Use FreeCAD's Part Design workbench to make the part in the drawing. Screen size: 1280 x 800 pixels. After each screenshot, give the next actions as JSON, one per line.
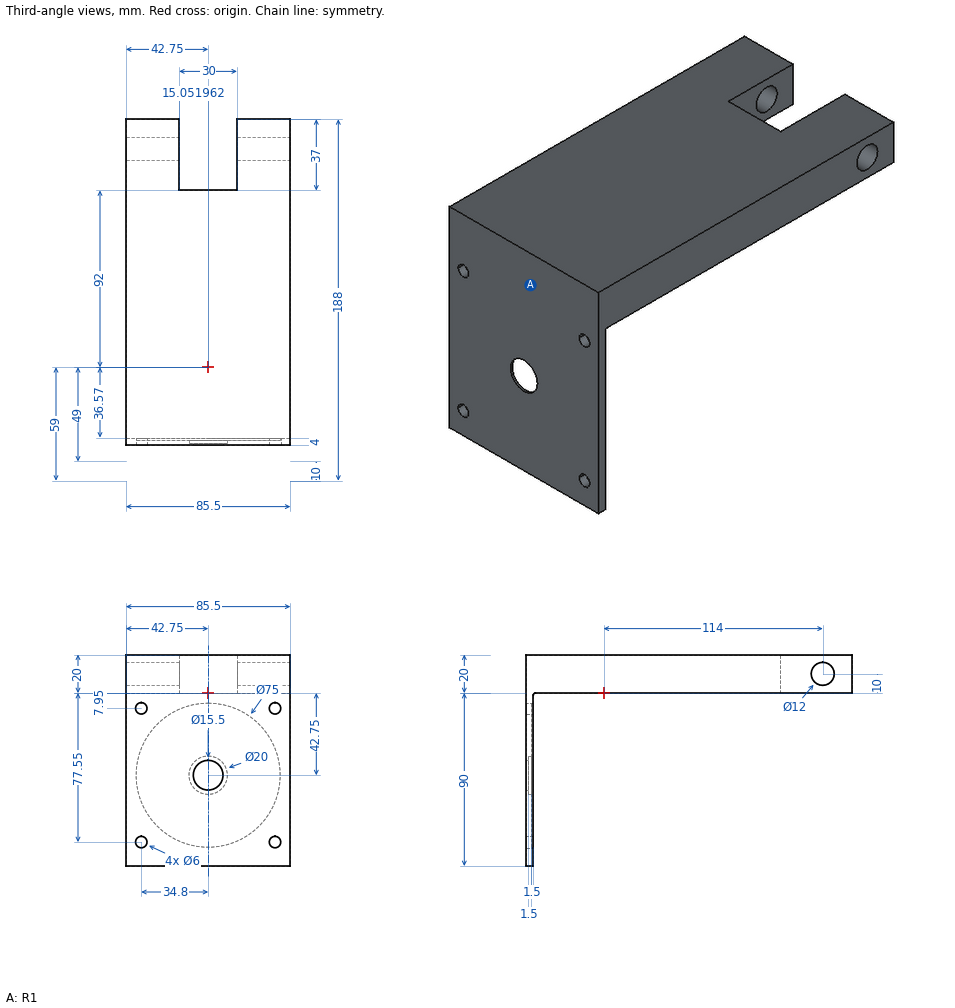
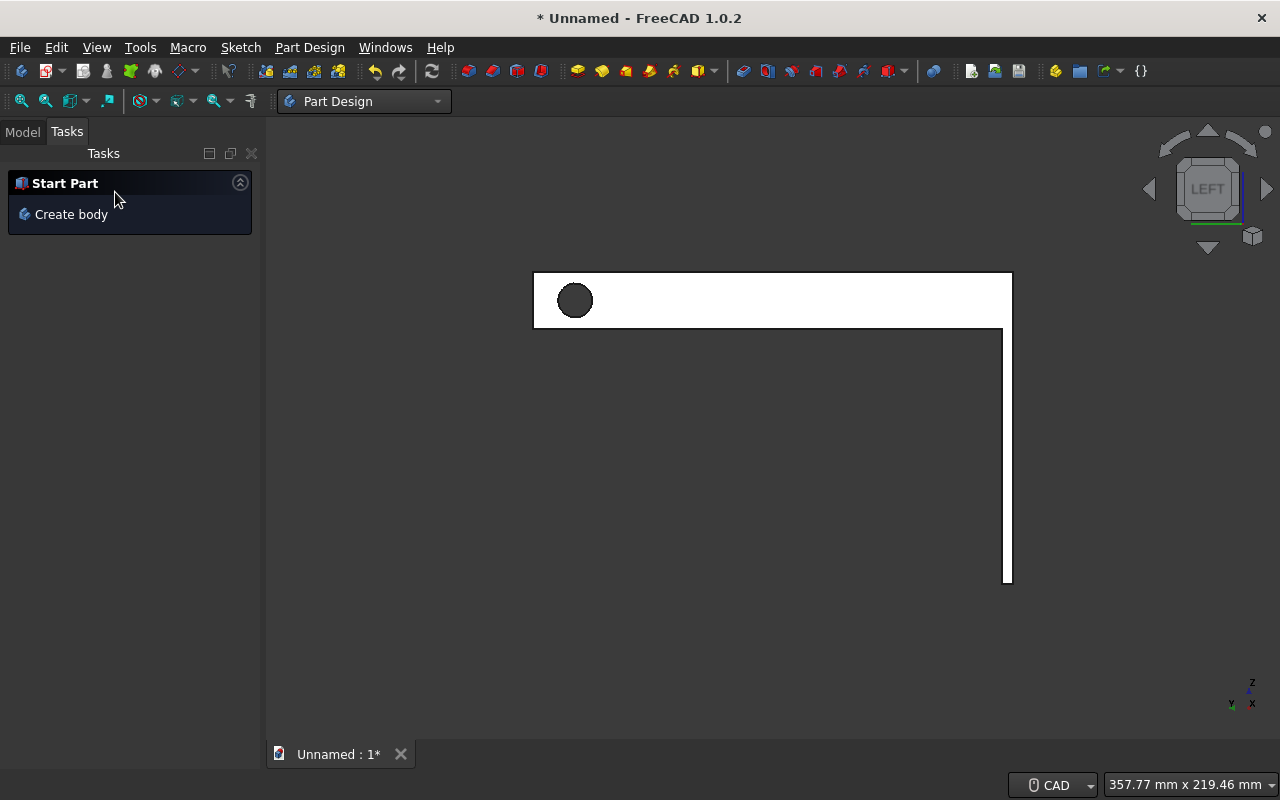
{"action": "key", "text": "v 3"}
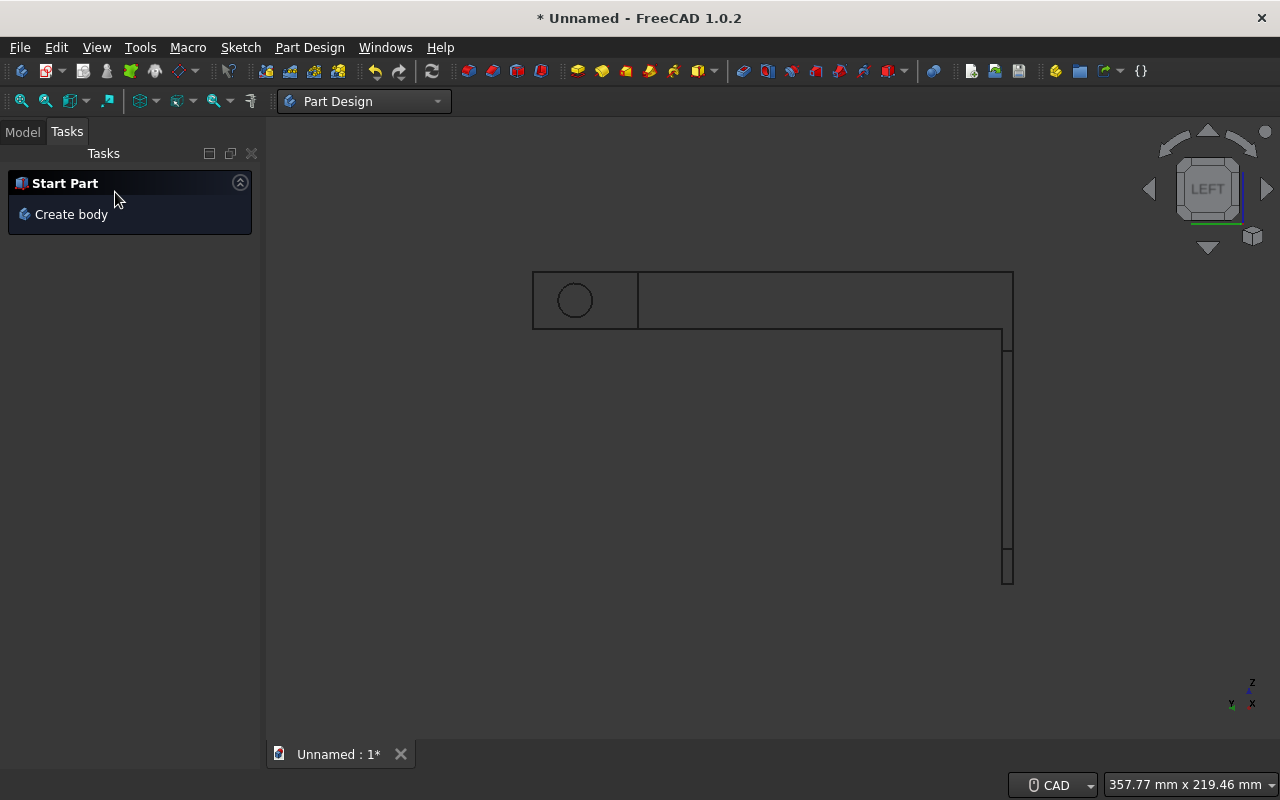
{"action": "key", "text": "0"}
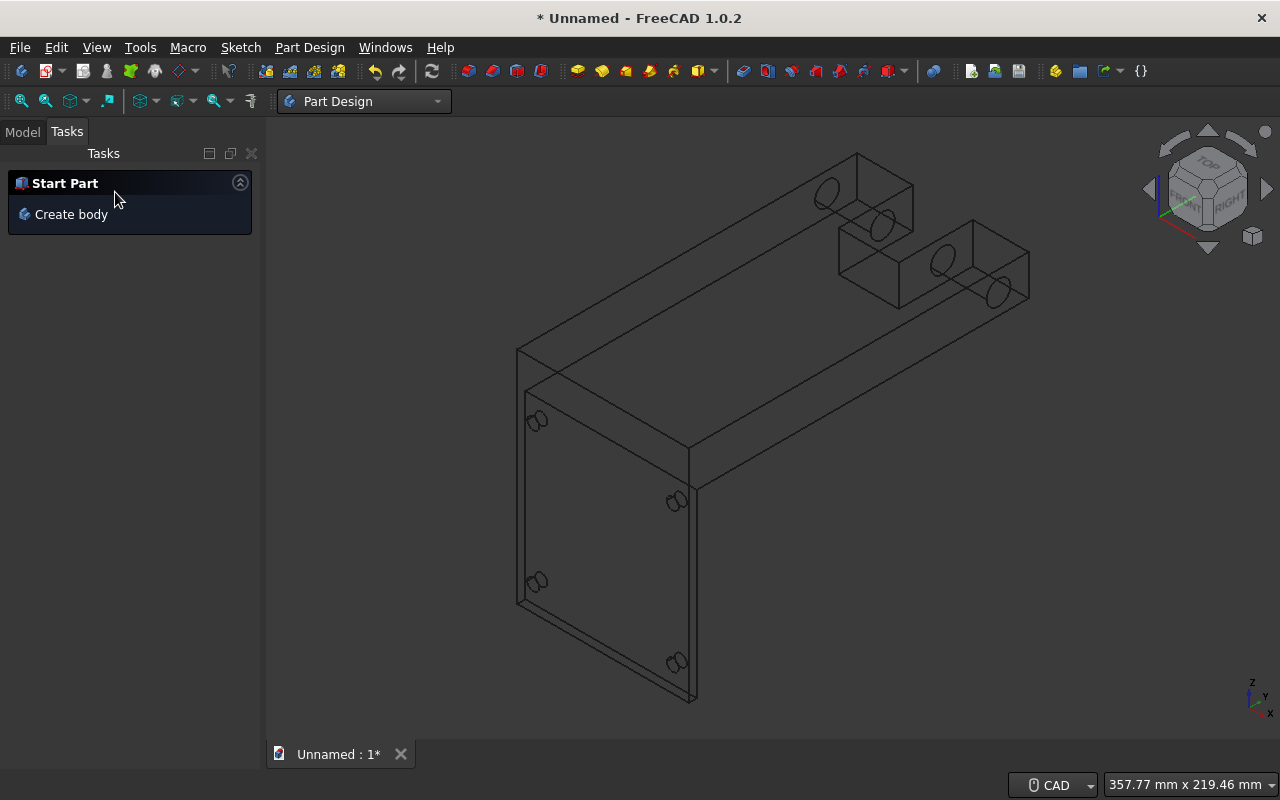
{"action": "left_click", "coordinate": [611, 439]}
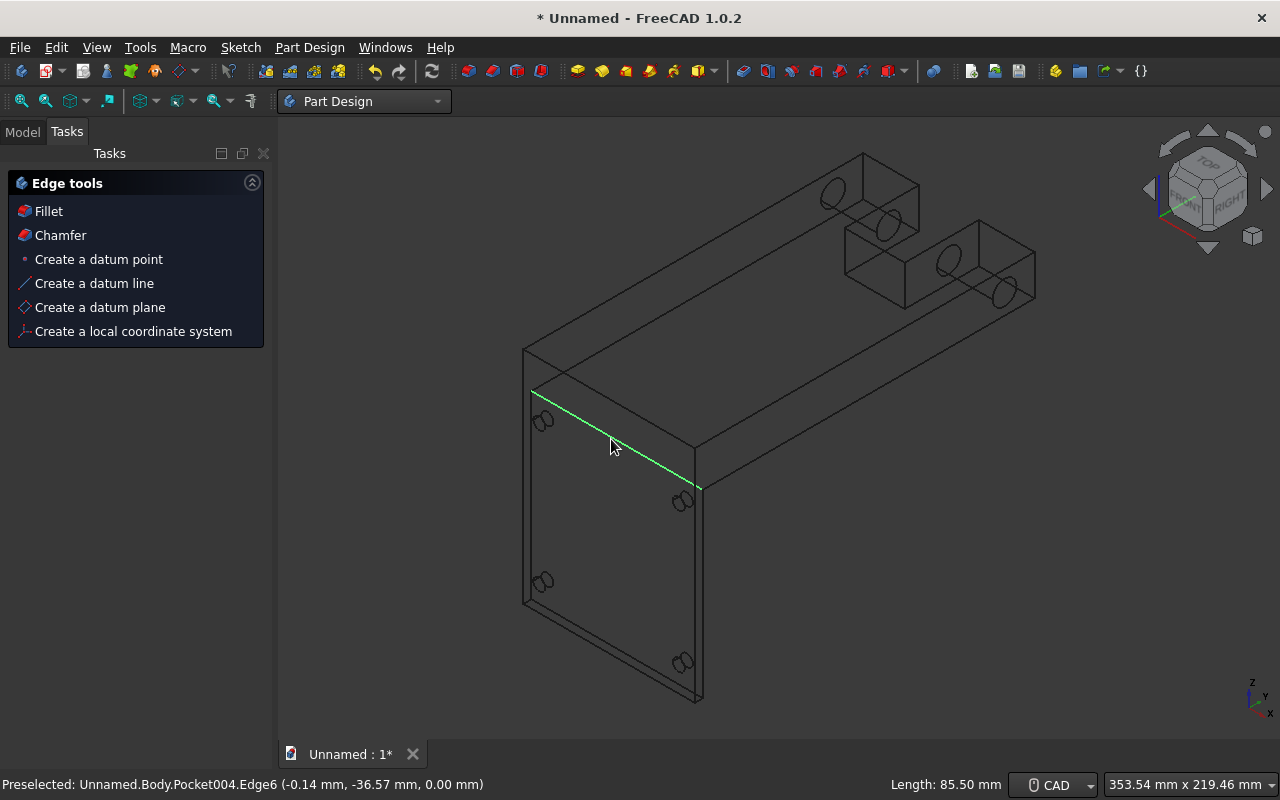
{"action": "key", "text": "v 1"}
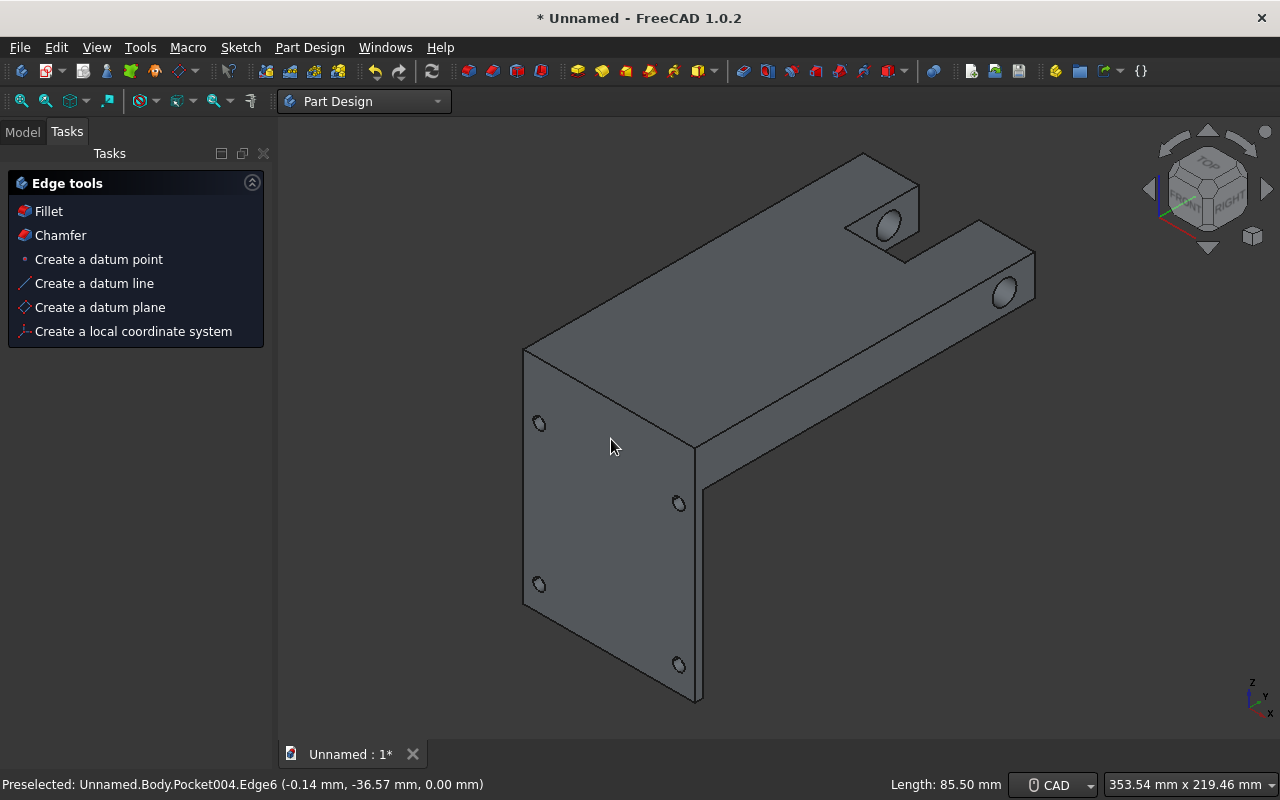
{"action": "left_click", "coordinate": [470, 72]}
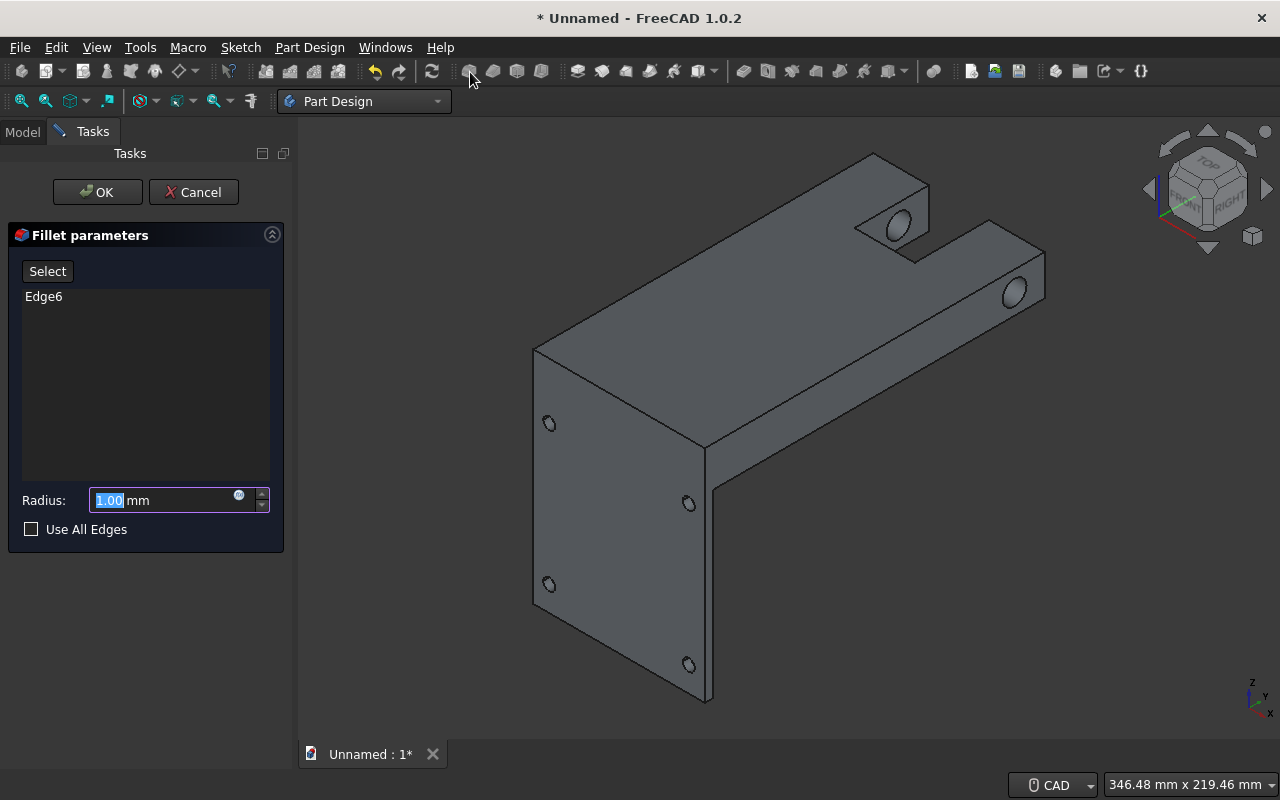
{"action": "type", "text": "1"}
{"action": "key", "text": "Tab"}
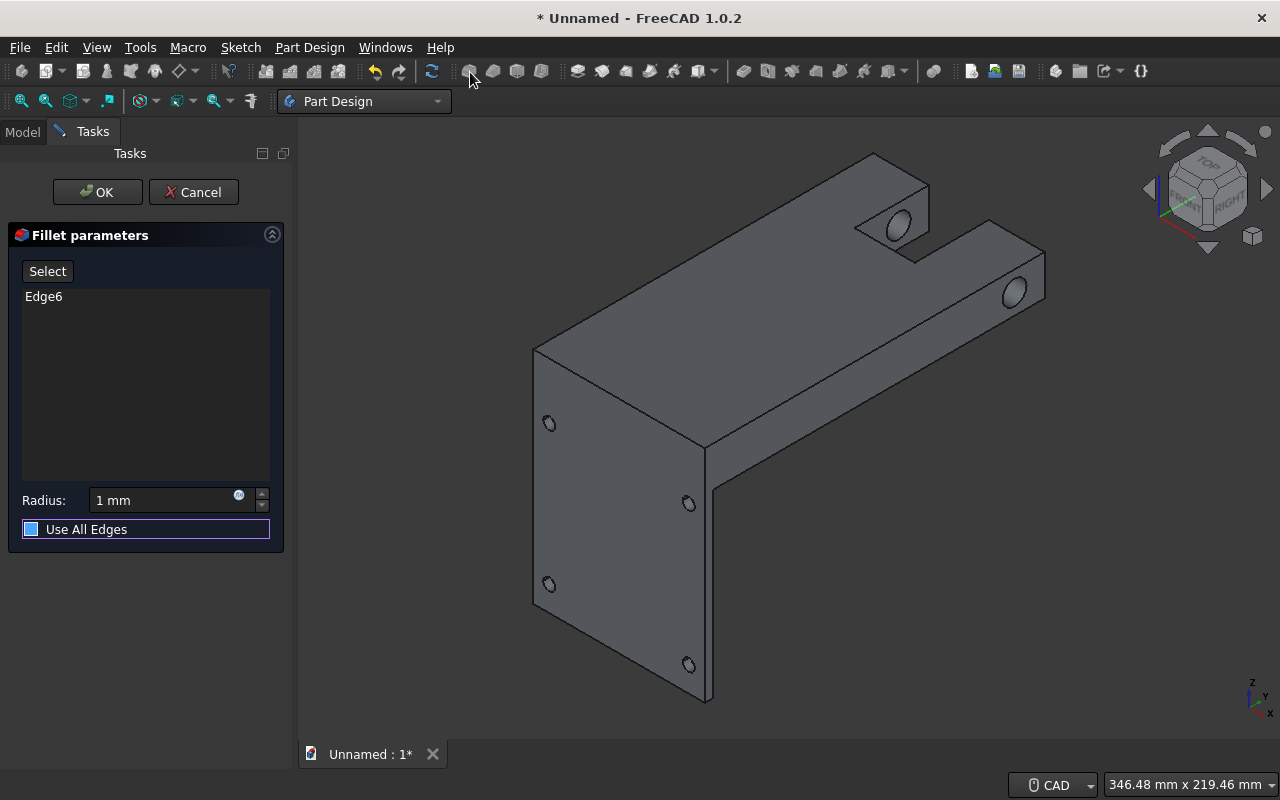
{"action": "left_click", "coordinate": [98, 192]}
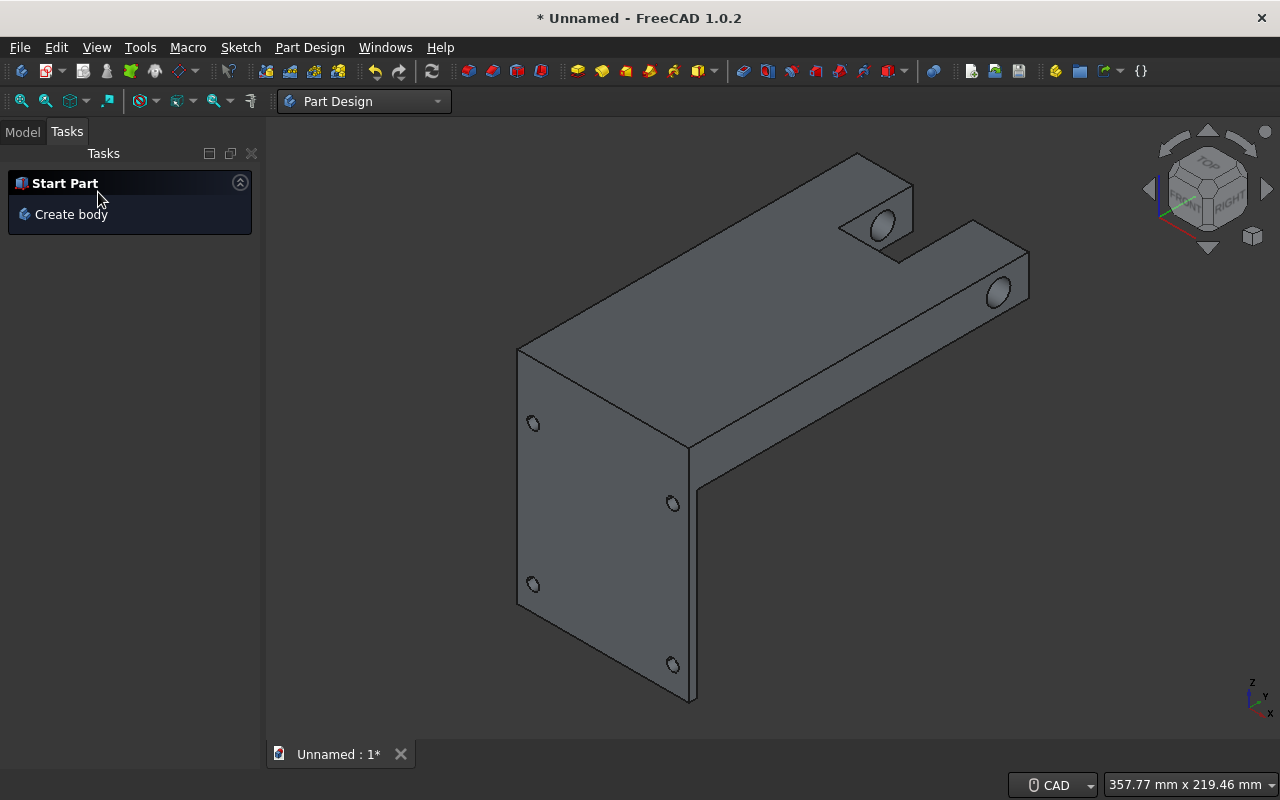
{"action": "key", "text": "4"}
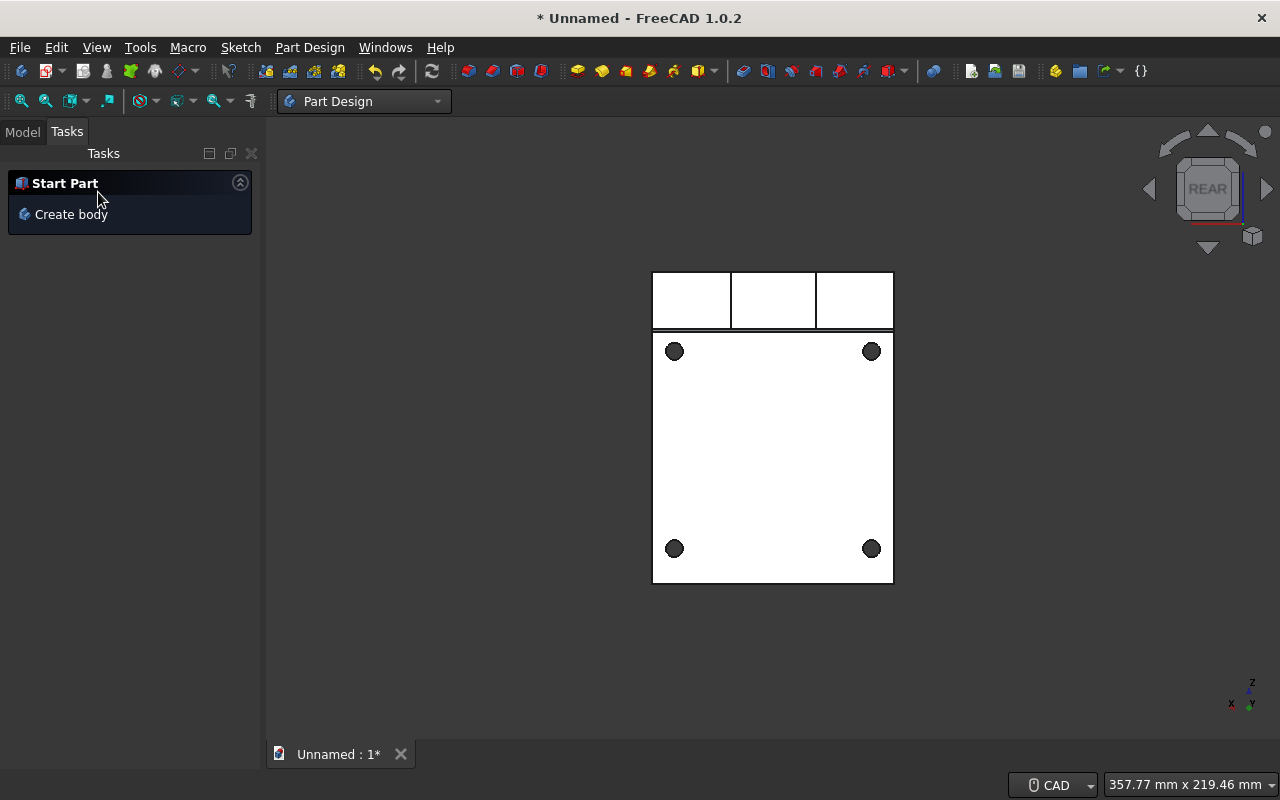
{"action": "left_click", "coordinate": [773, 457]}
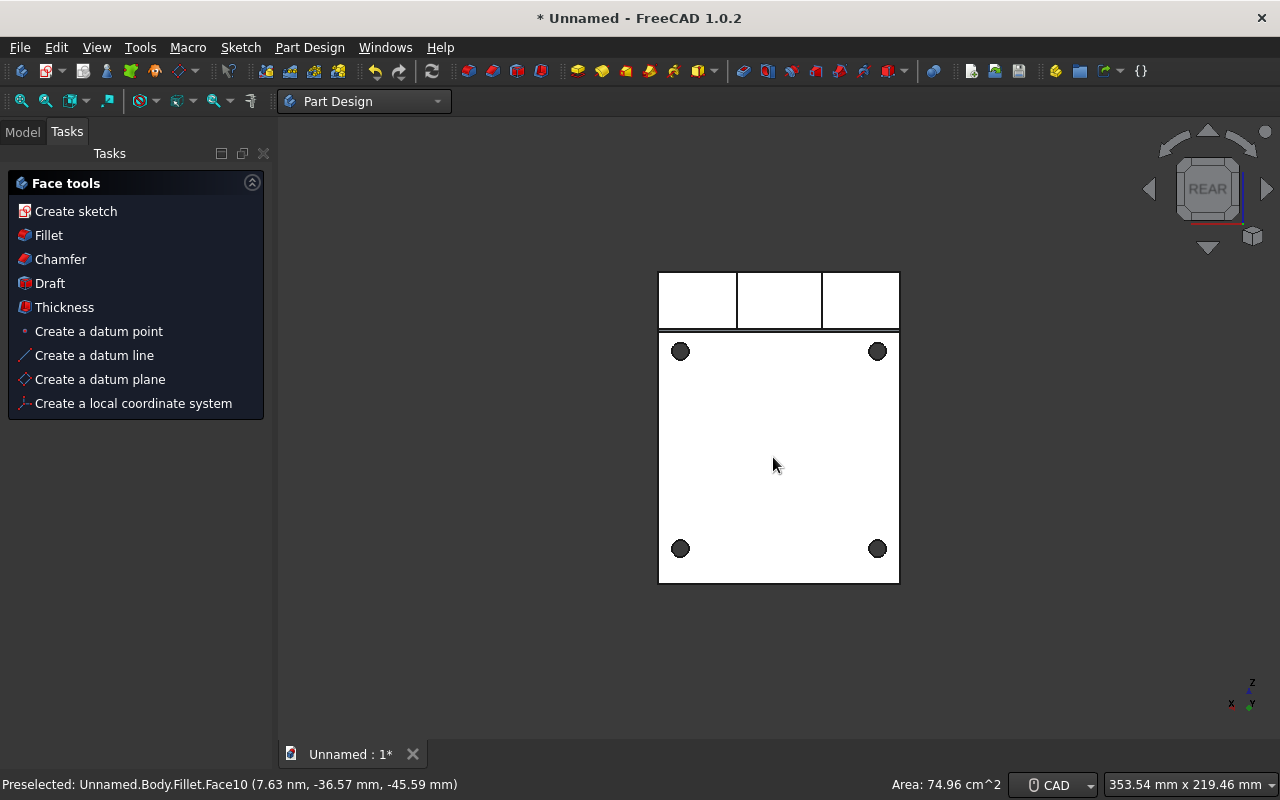
{"action": "left_click", "coordinate": [46, 72]}